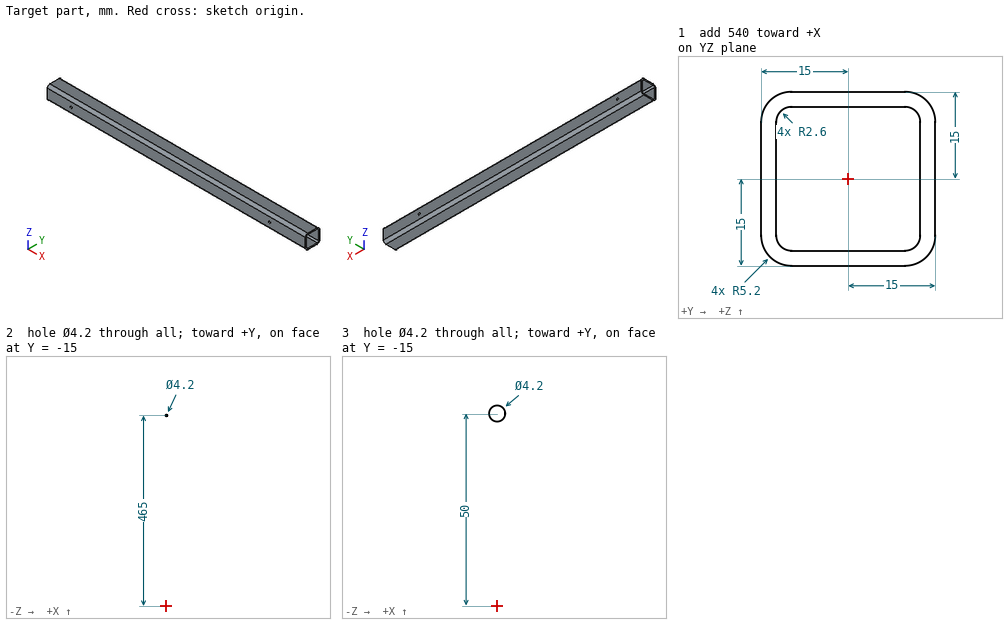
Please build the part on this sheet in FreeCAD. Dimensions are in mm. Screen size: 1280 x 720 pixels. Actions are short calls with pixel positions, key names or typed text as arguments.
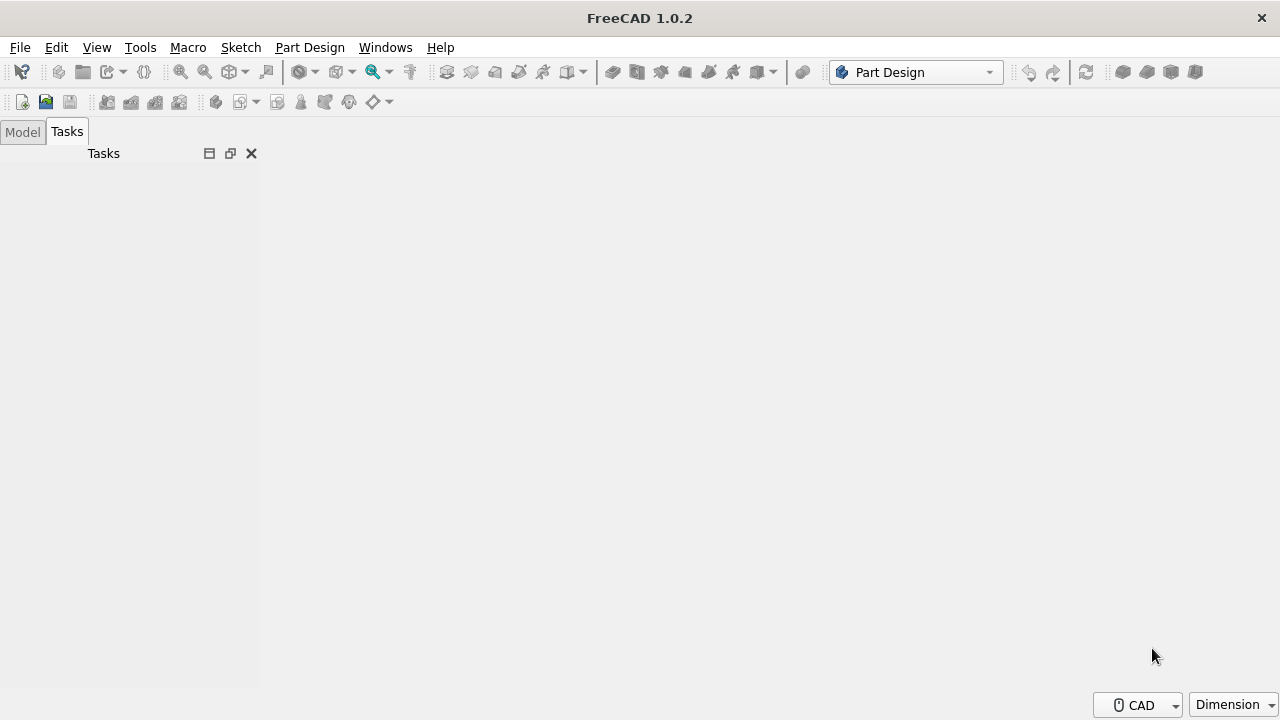
click(22, 102)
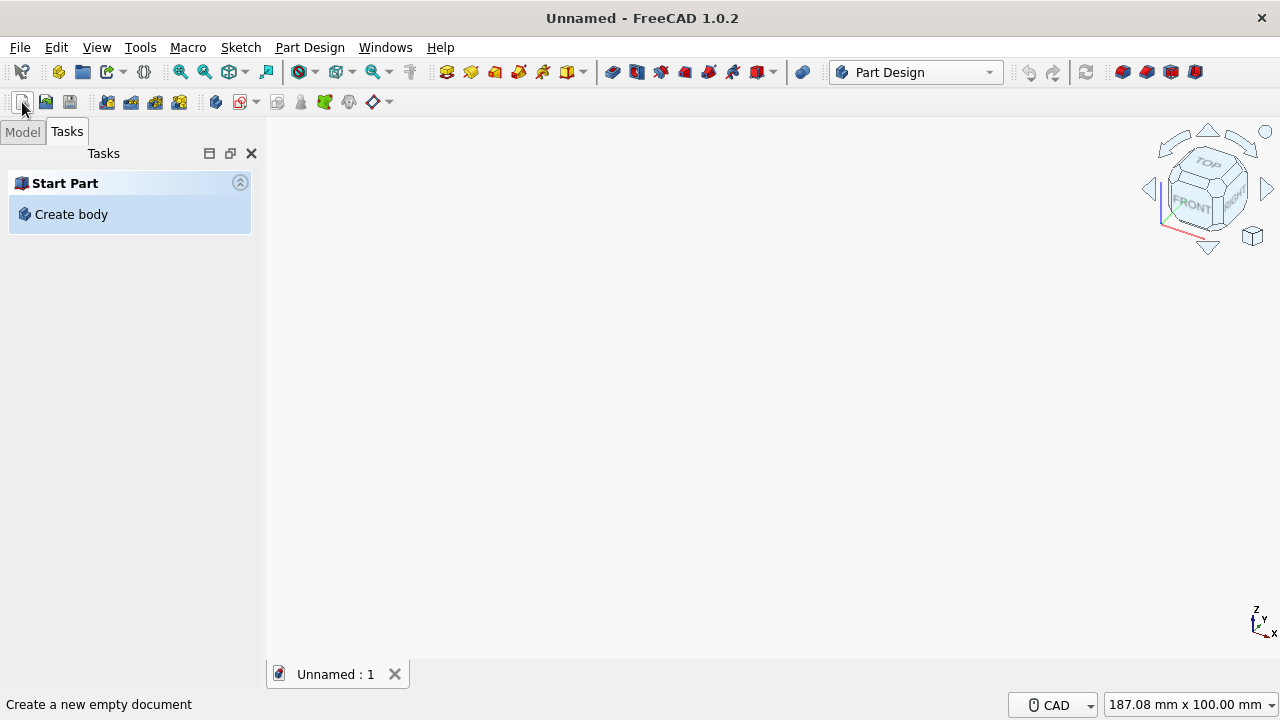
click(240, 102)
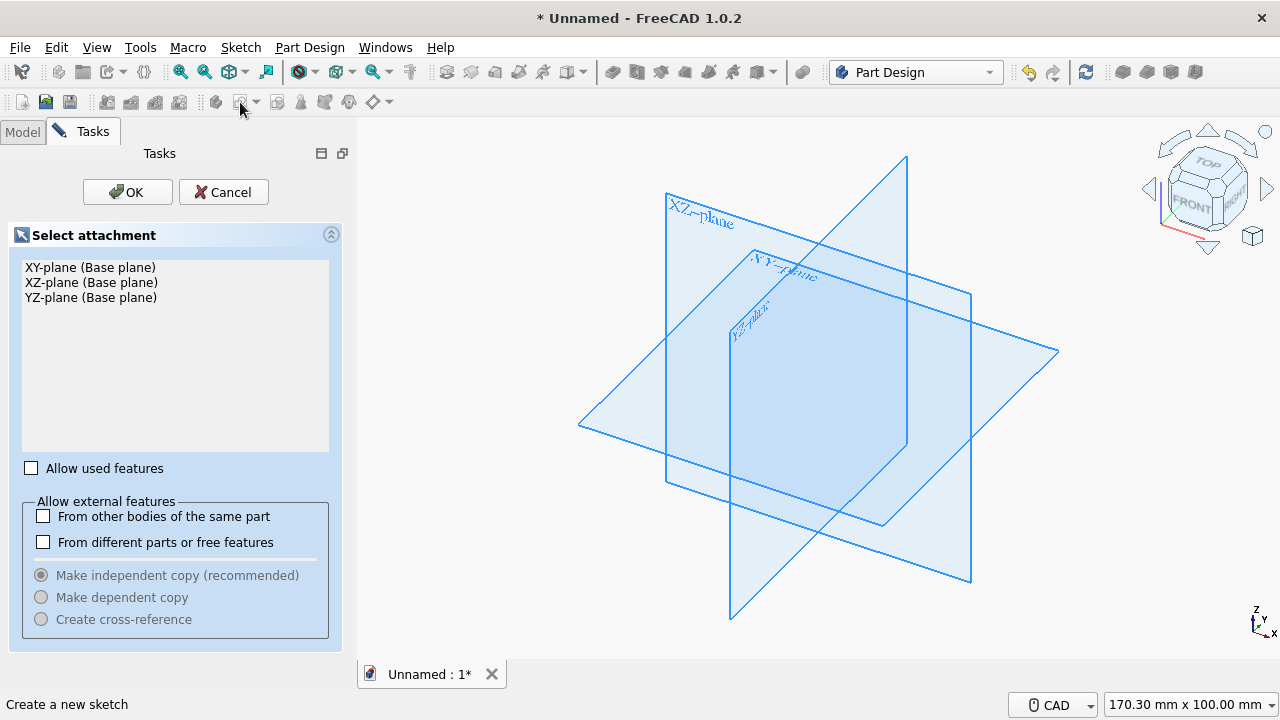
click(82, 298)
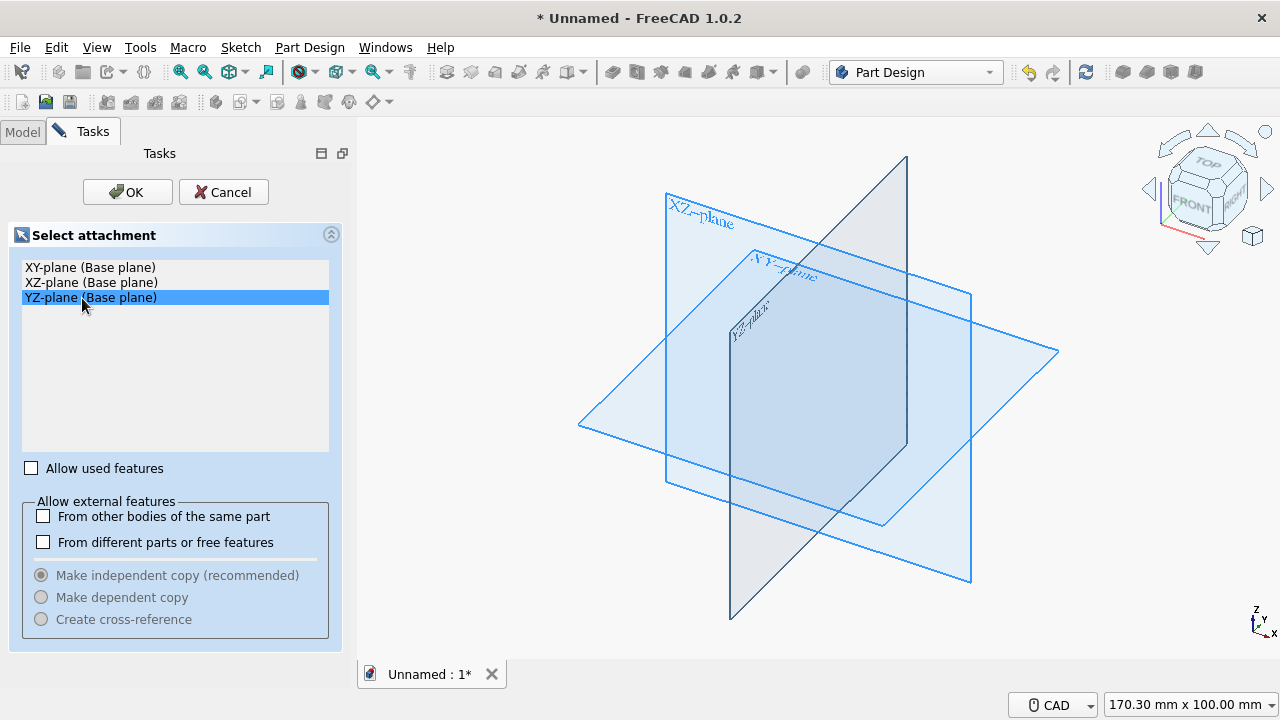
click(128, 192)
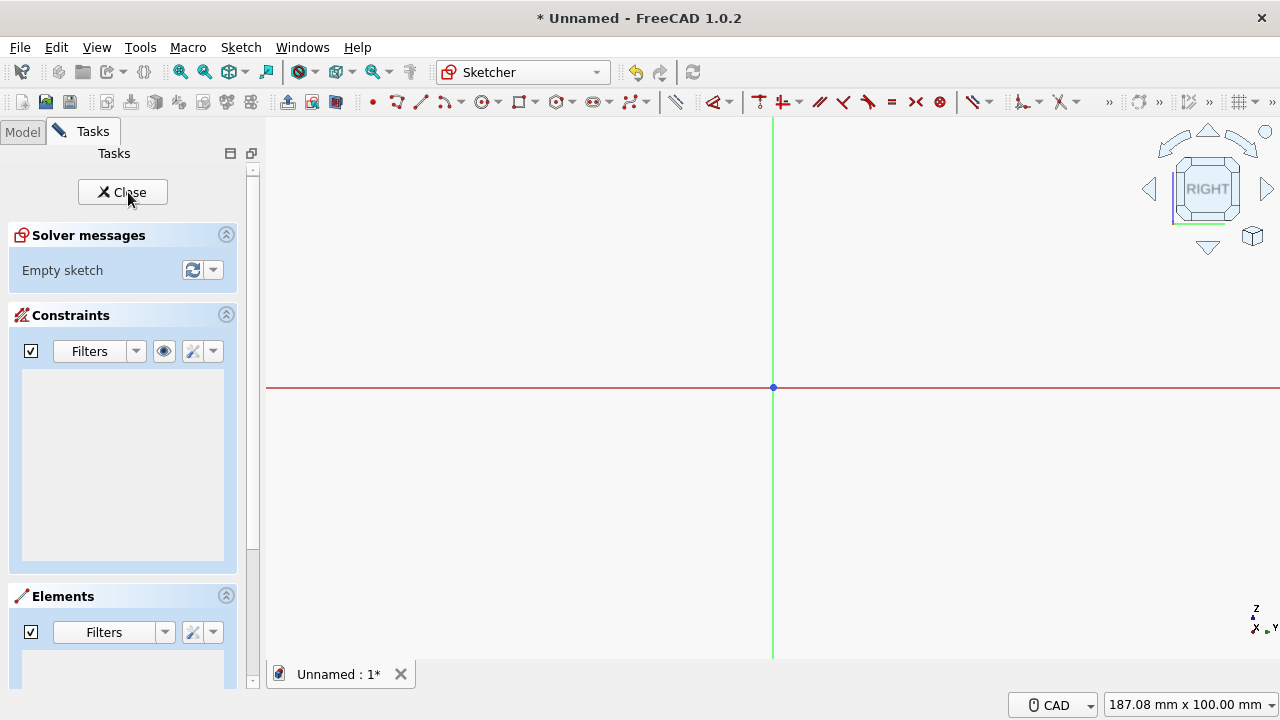
scroll(829, 388, up, 4)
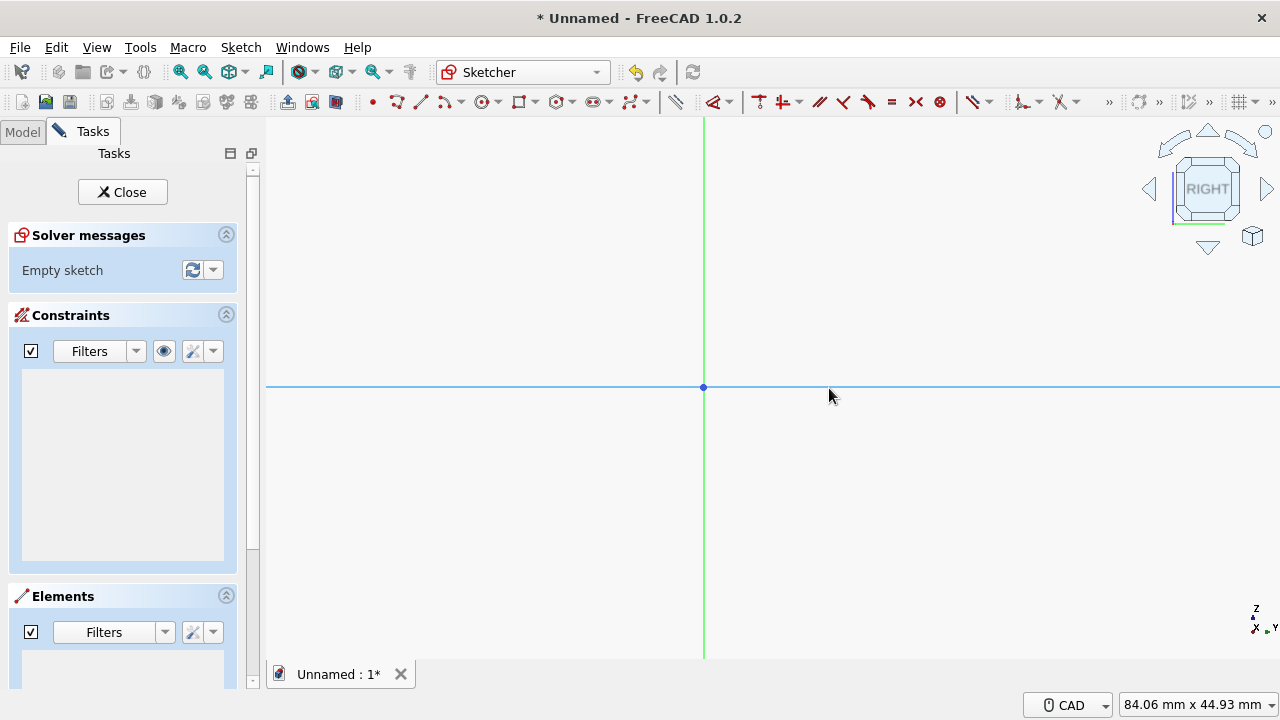
click(422, 102)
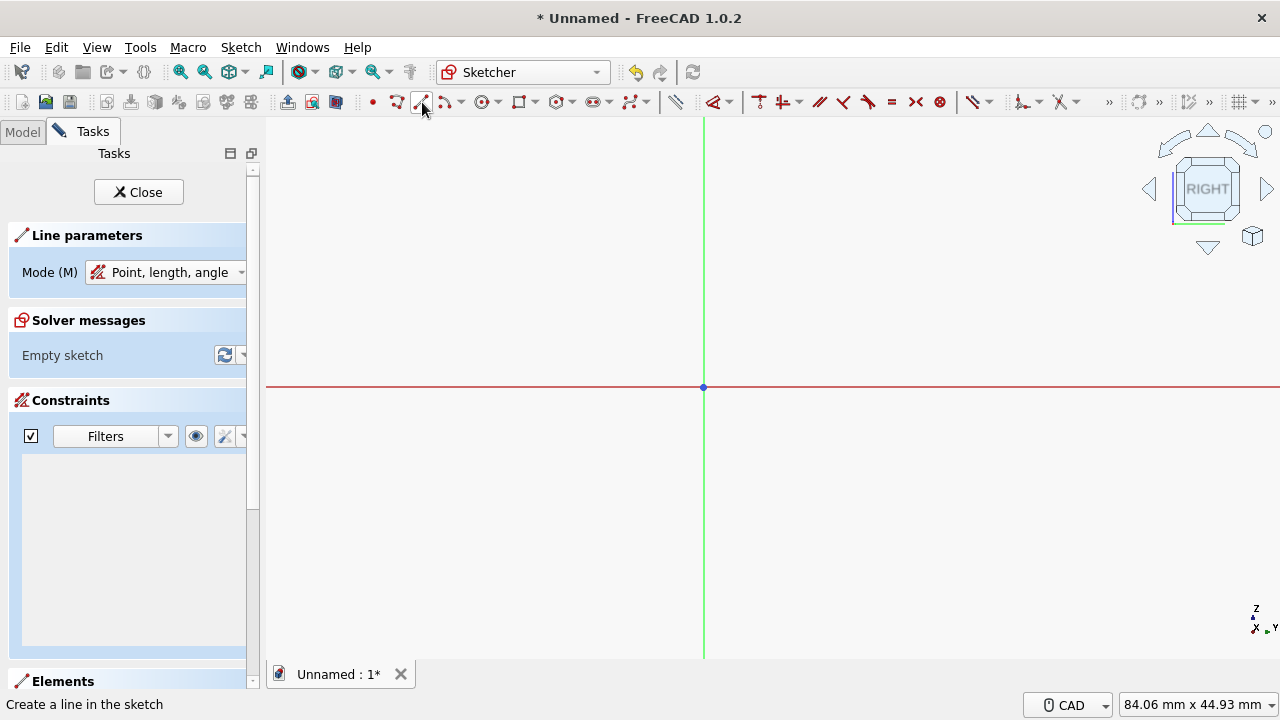
click(523, 269)
click(523, 506)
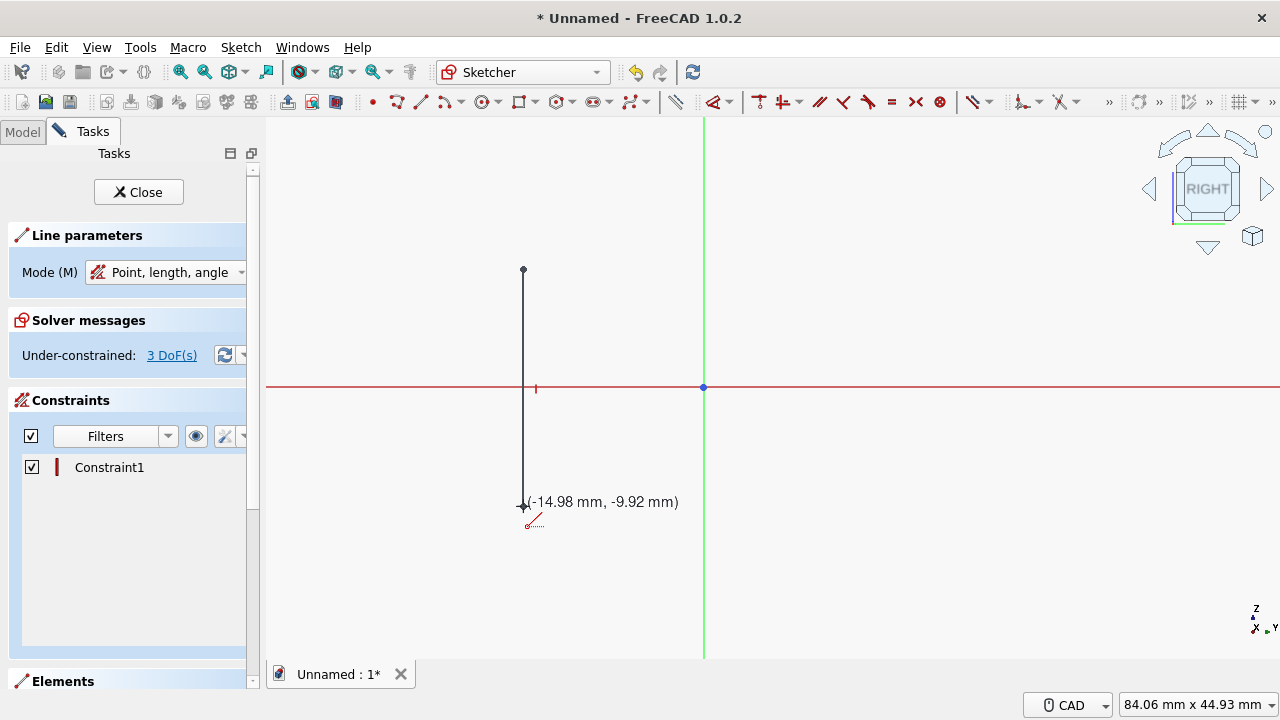
click(585, 568)
click(822, 568)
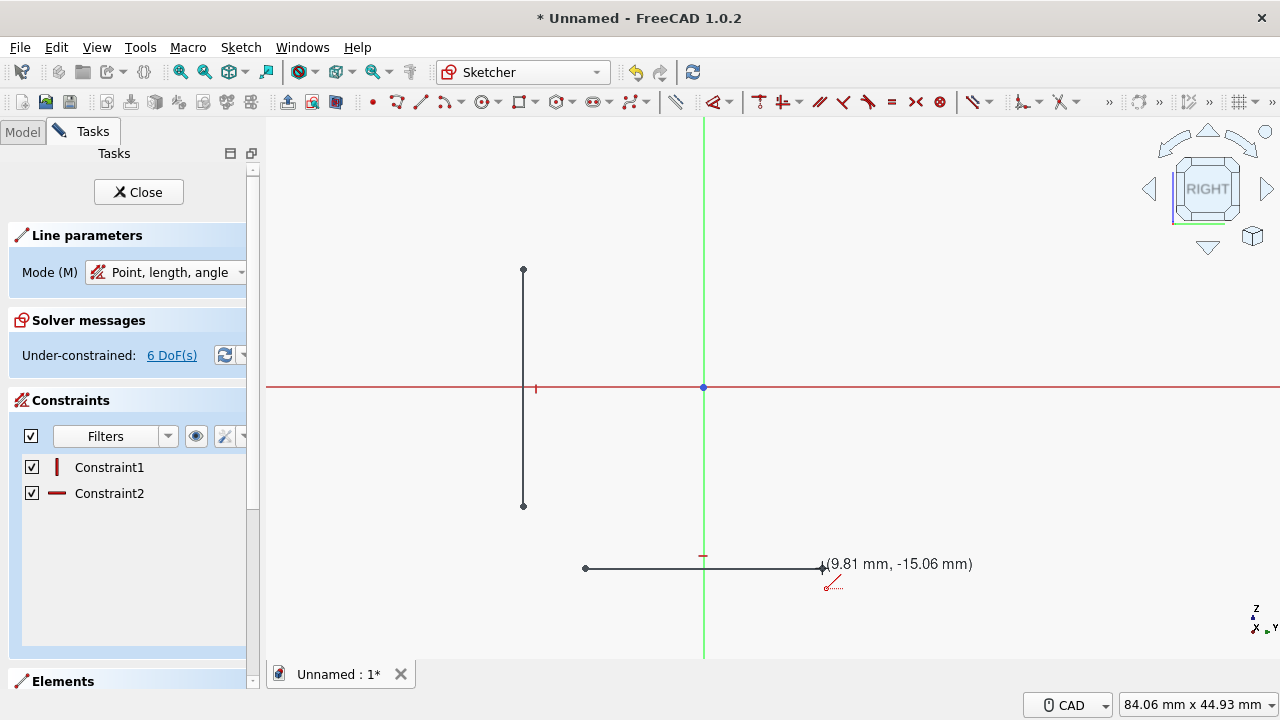
click(885, 506)
click(885, 269)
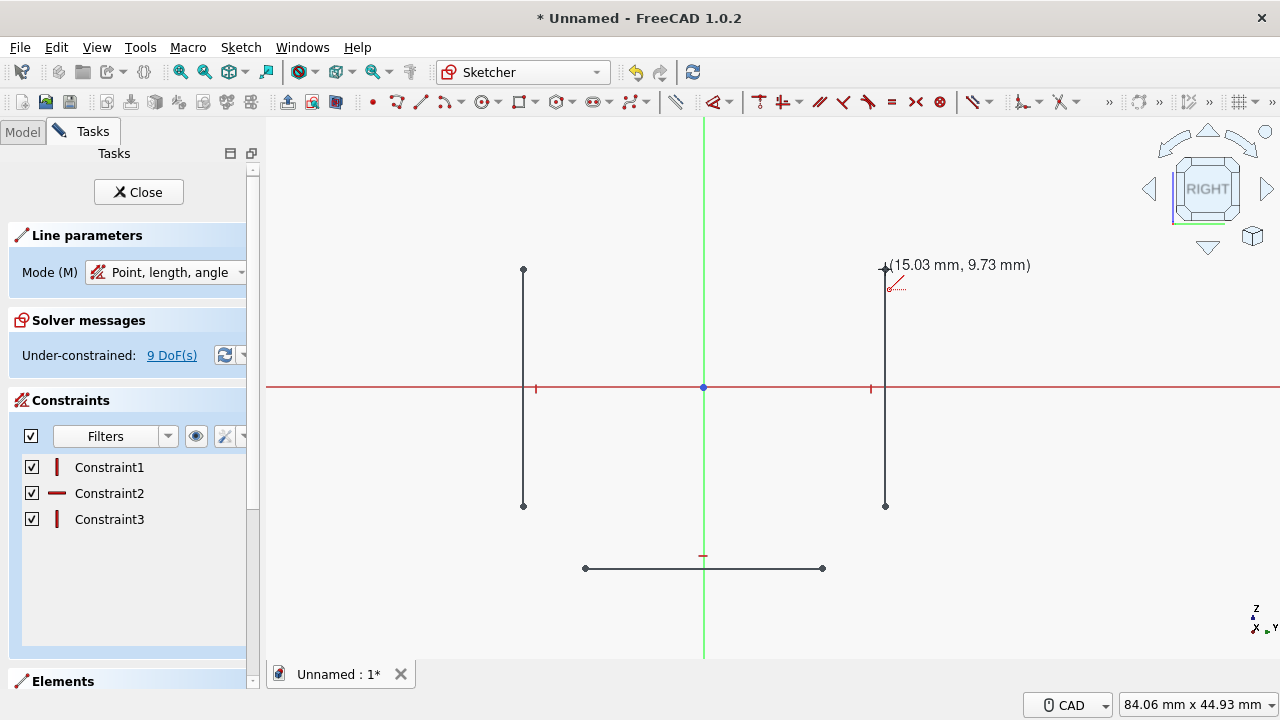
click(822, 206)
click(585, 206)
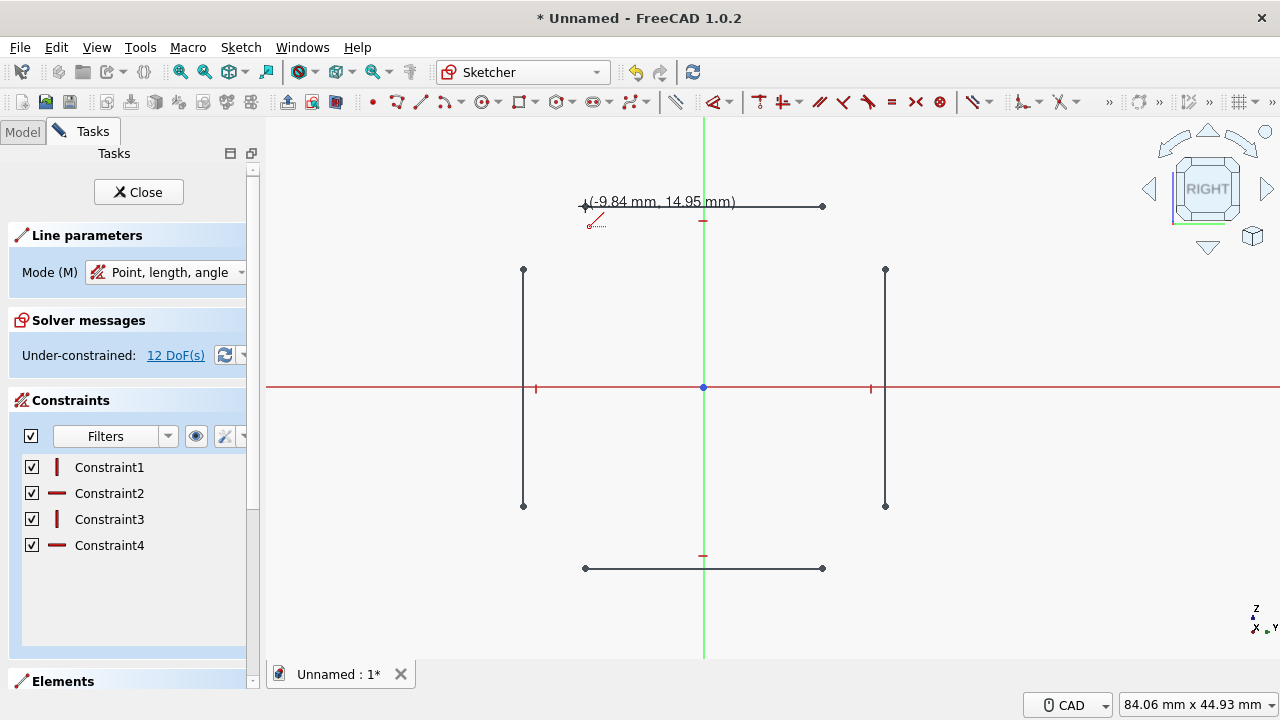
key(g)
key(3)
key(a)